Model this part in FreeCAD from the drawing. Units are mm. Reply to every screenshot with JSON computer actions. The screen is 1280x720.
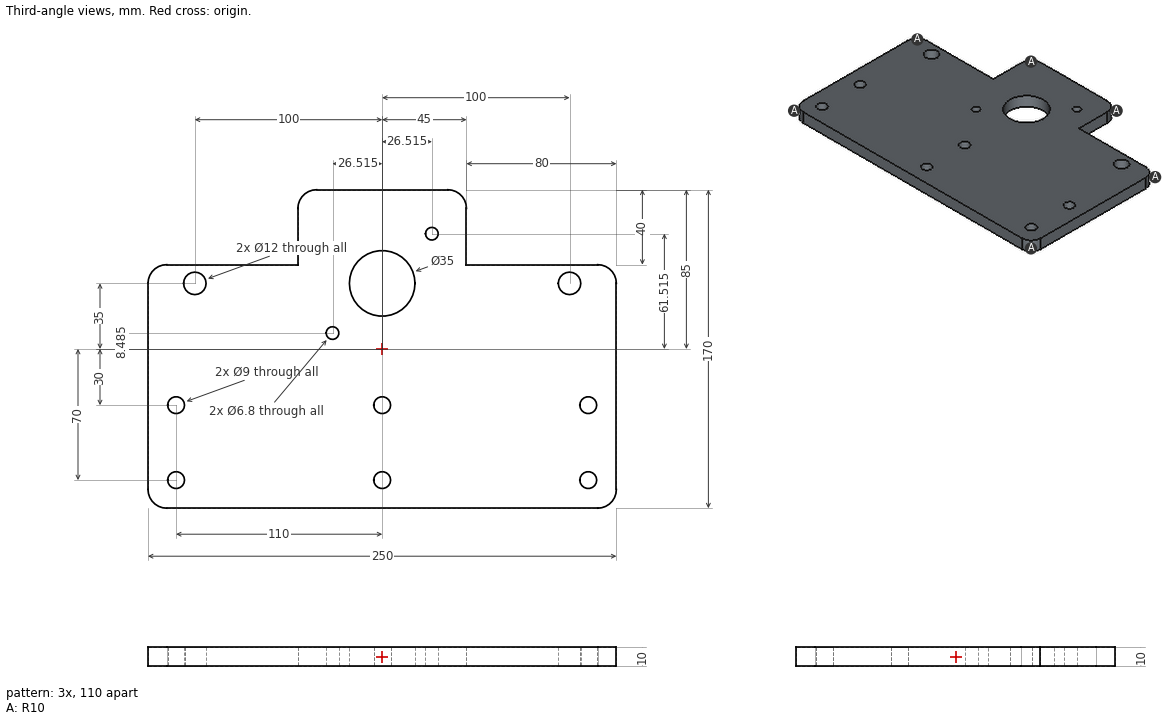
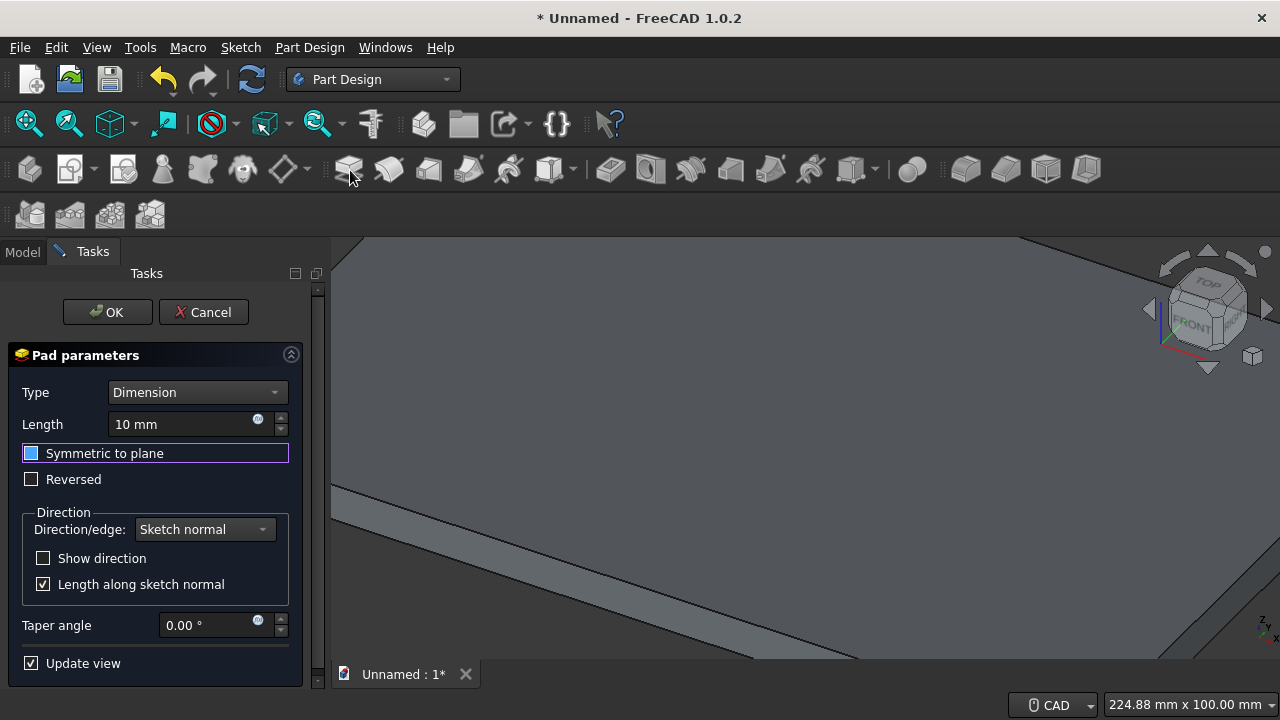
{"action": "left_click", "coordinate": [30, 453]}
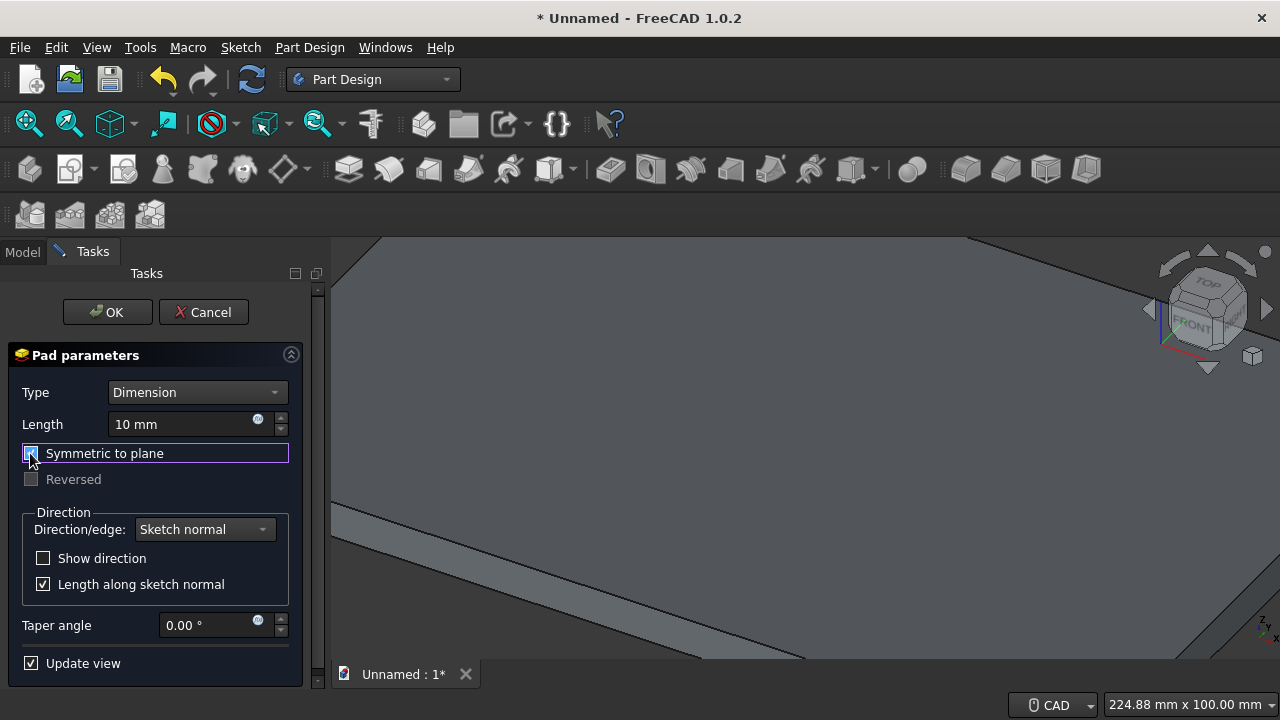
{"action": "left_click", "coordinate": [108, 312]}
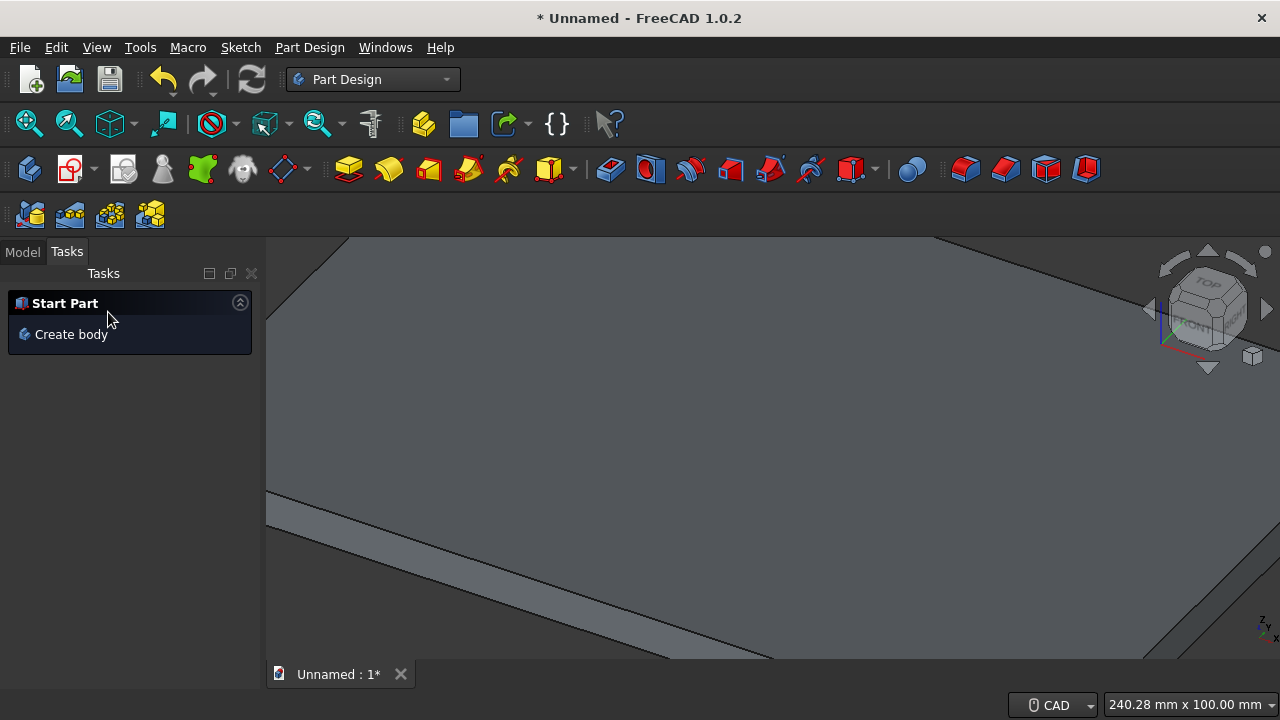
{"action": "left_click", "coordinate": [30, 124]}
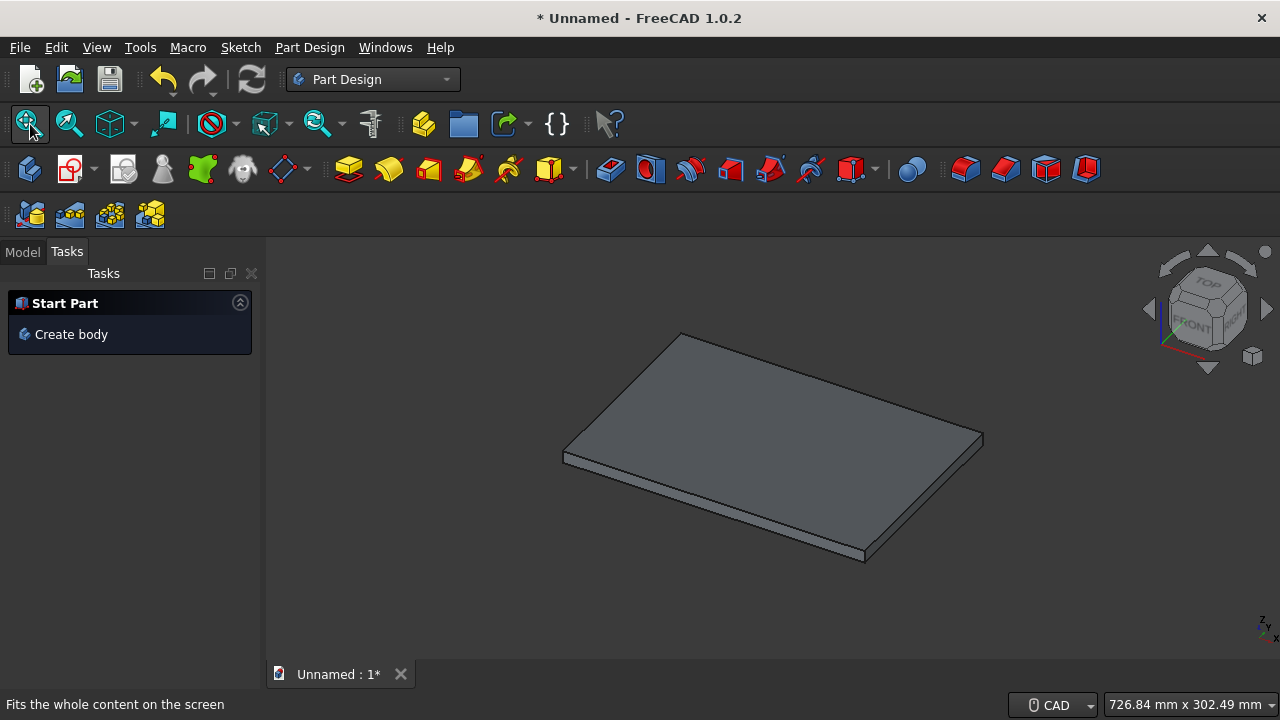
{"action": "left_click", "coordinate": [816, 456]}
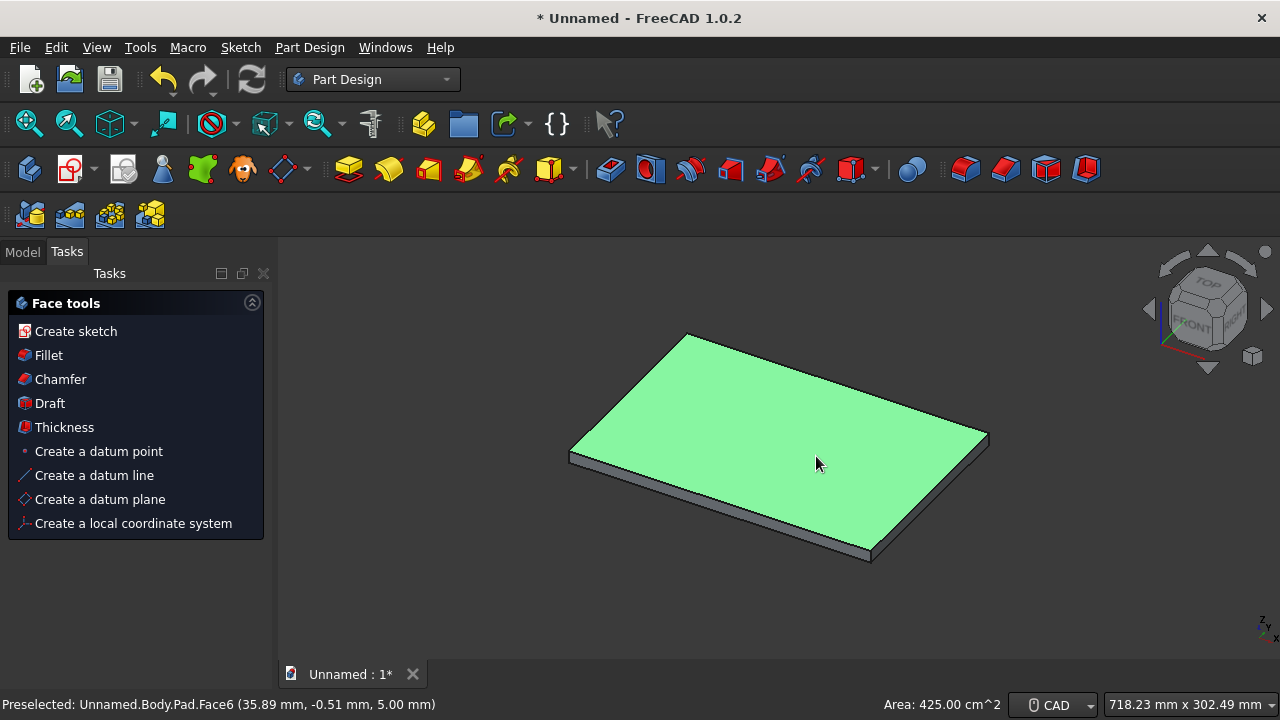
{"action": "left_click", "coordinate": [70, 170]}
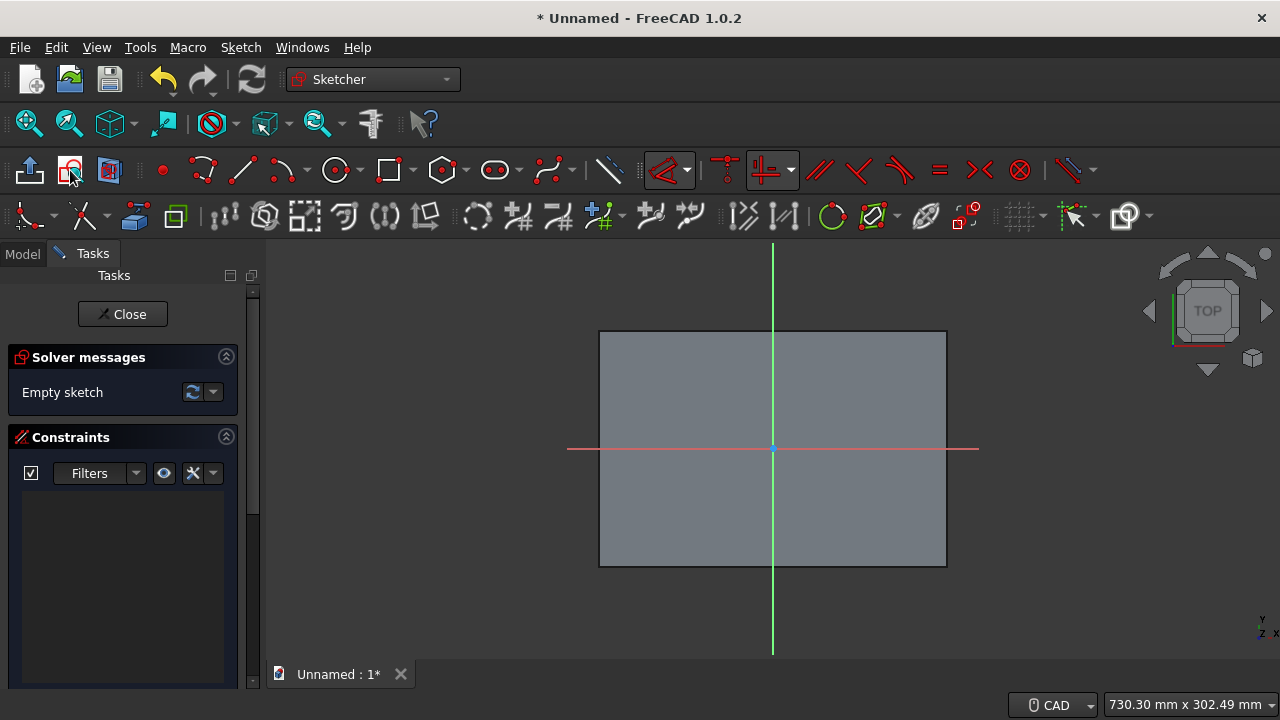
{"action": "scroll", "coordinate": [986, 342], "scroll_direction": "up", "scroll_amount": 4}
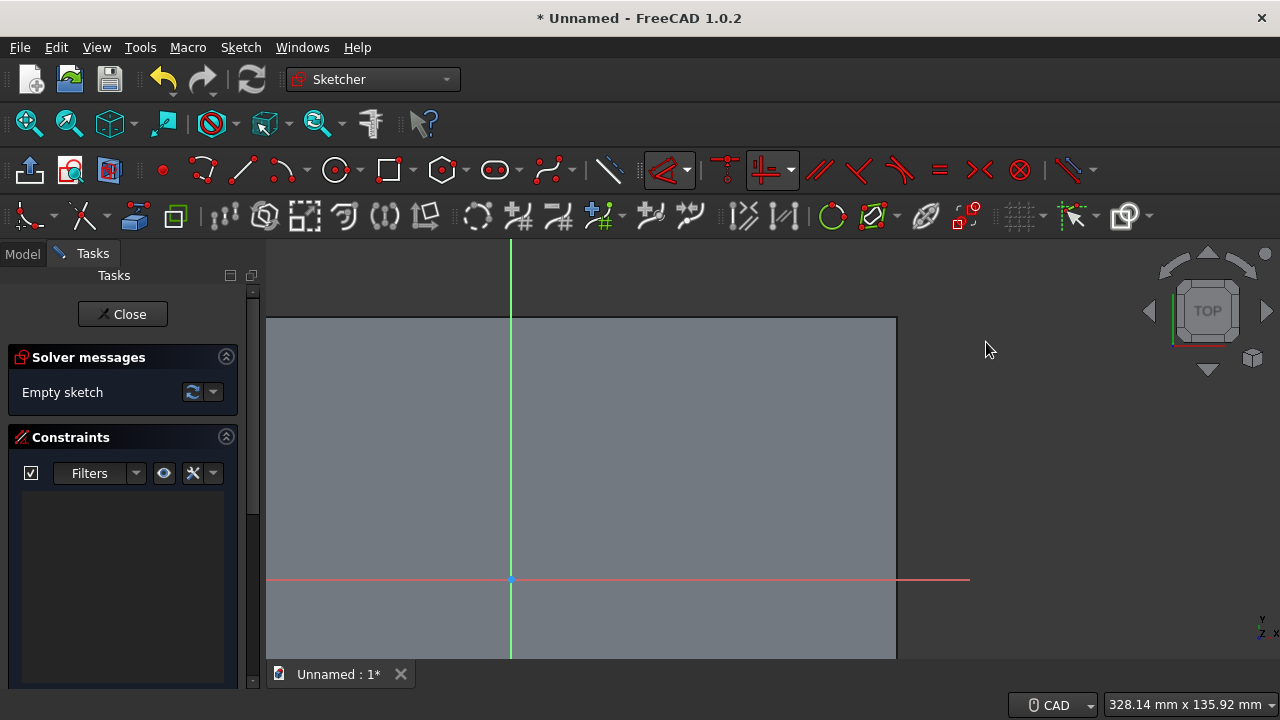
{"action": "left_click", "coordinate": [390, 170]}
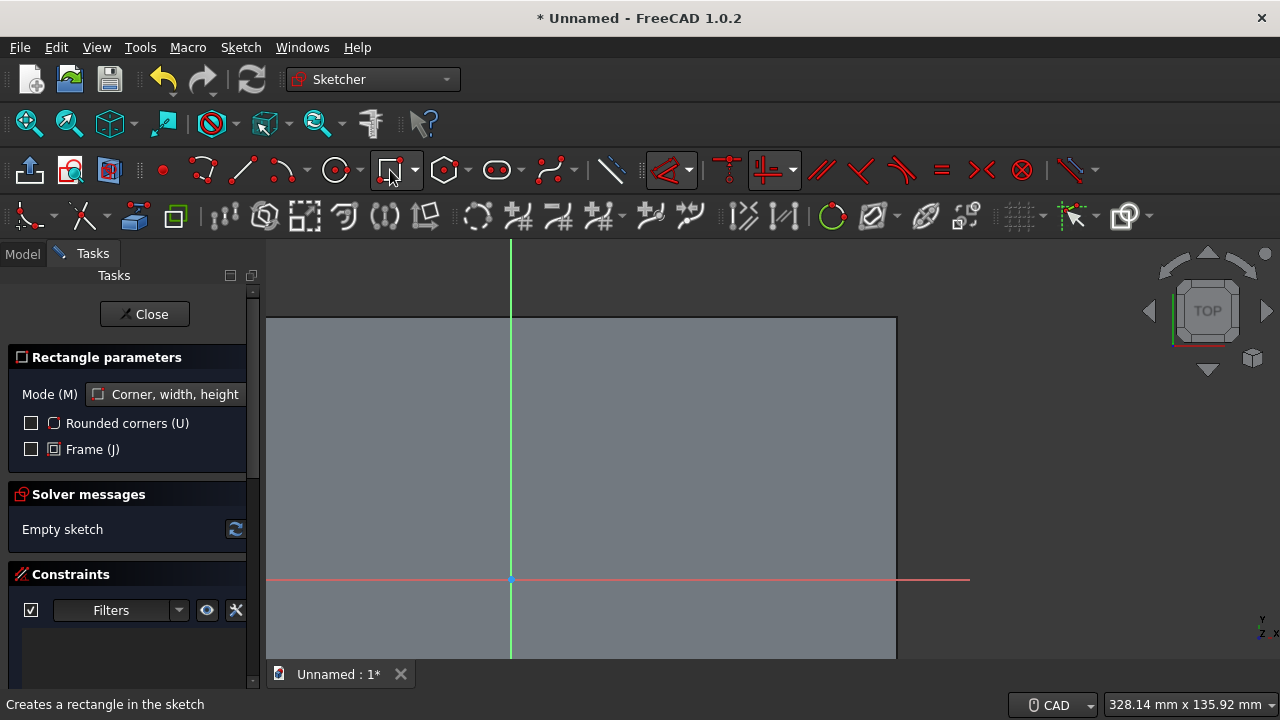
{"action": "left_click", "coordinate": [650, 317]}
{"action": "mouse_move", "coordinate": [897, 441]}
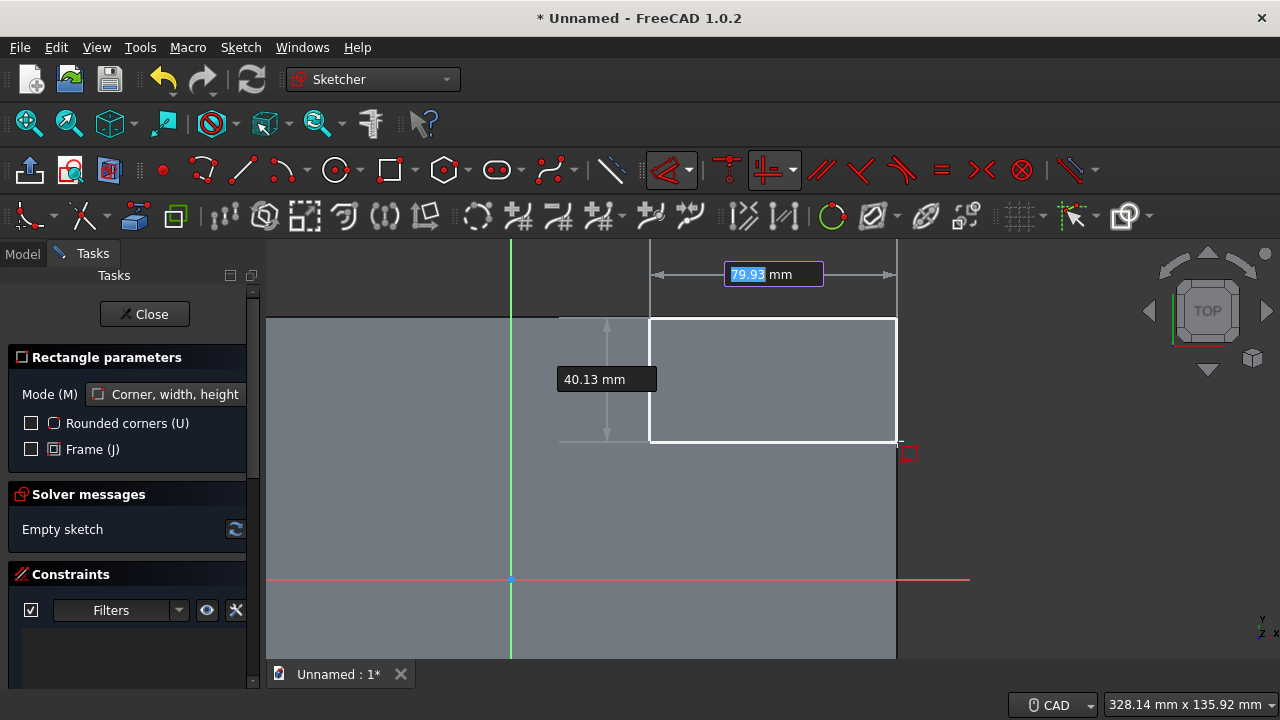
{"action": "type", "text": "80"}
{"action": "key", "text": "Tab"}
{"action": "type", "text": "40"}
{"action": "key", "text": "Return"}
{"action": "key", "text": "Escape"}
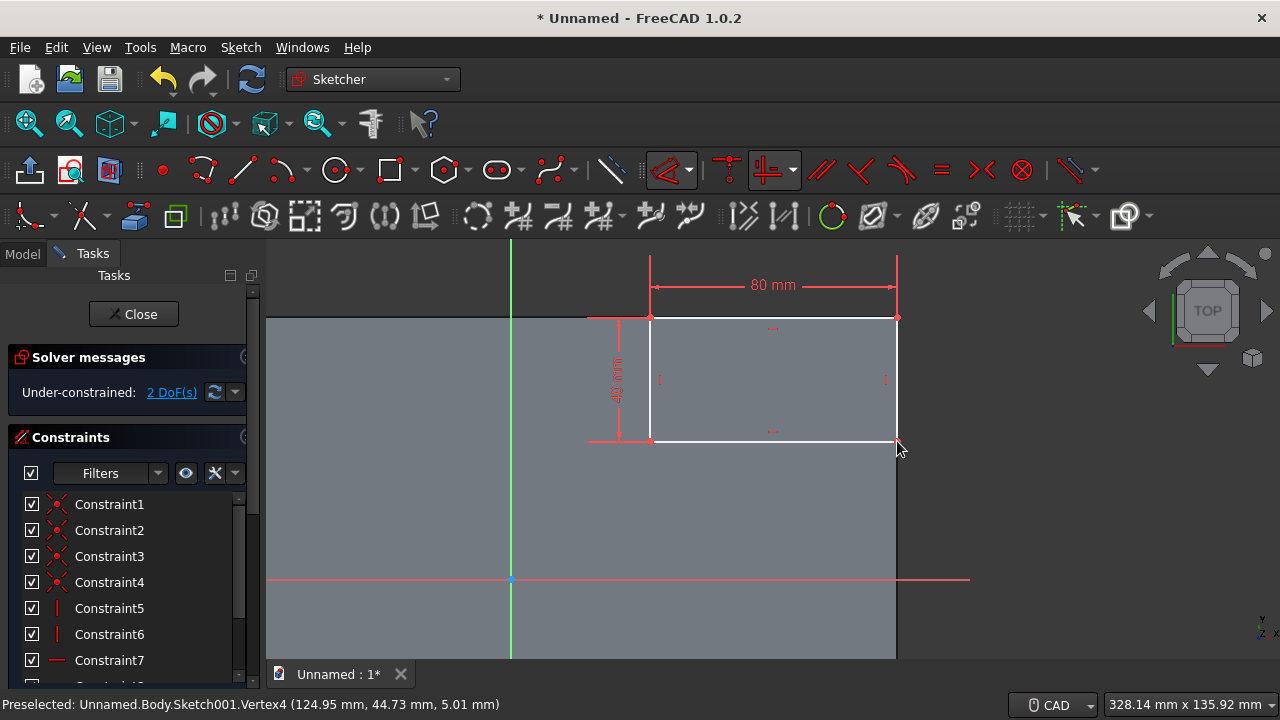
{"action": "left_click", "coordinate": [650, 318]}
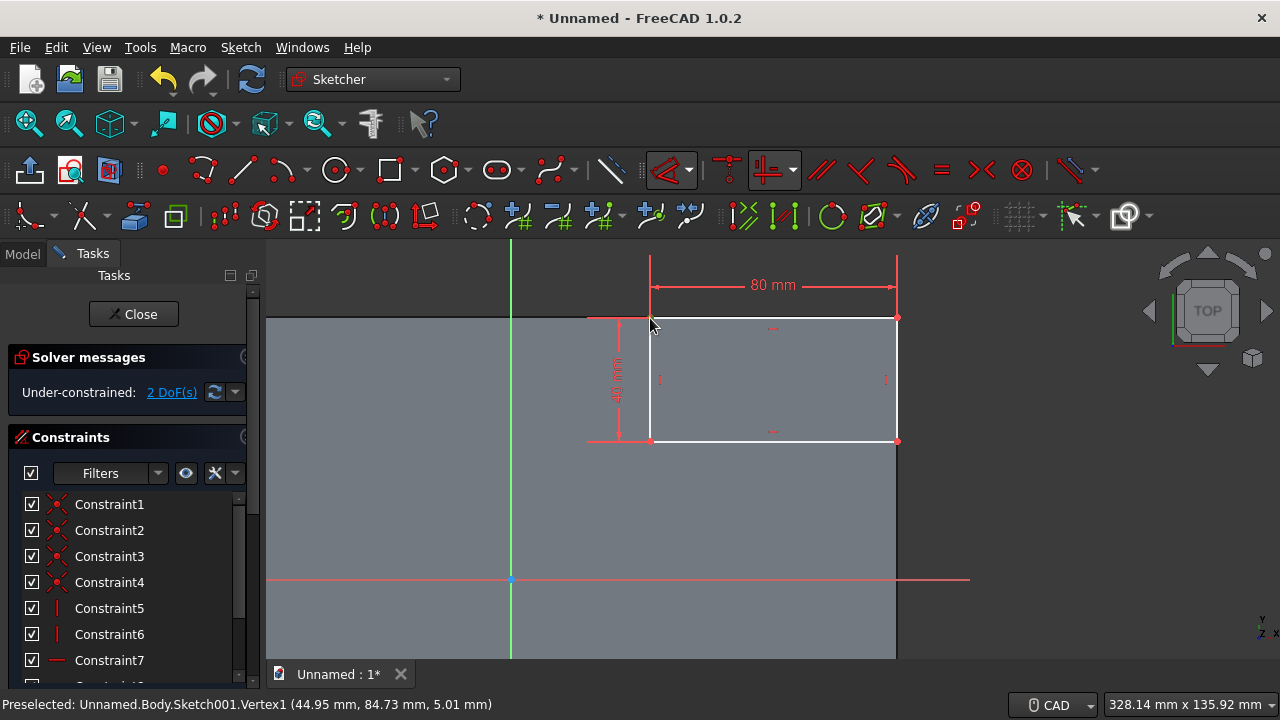
{"action": "left_click", "coordinate": [692, 170]}